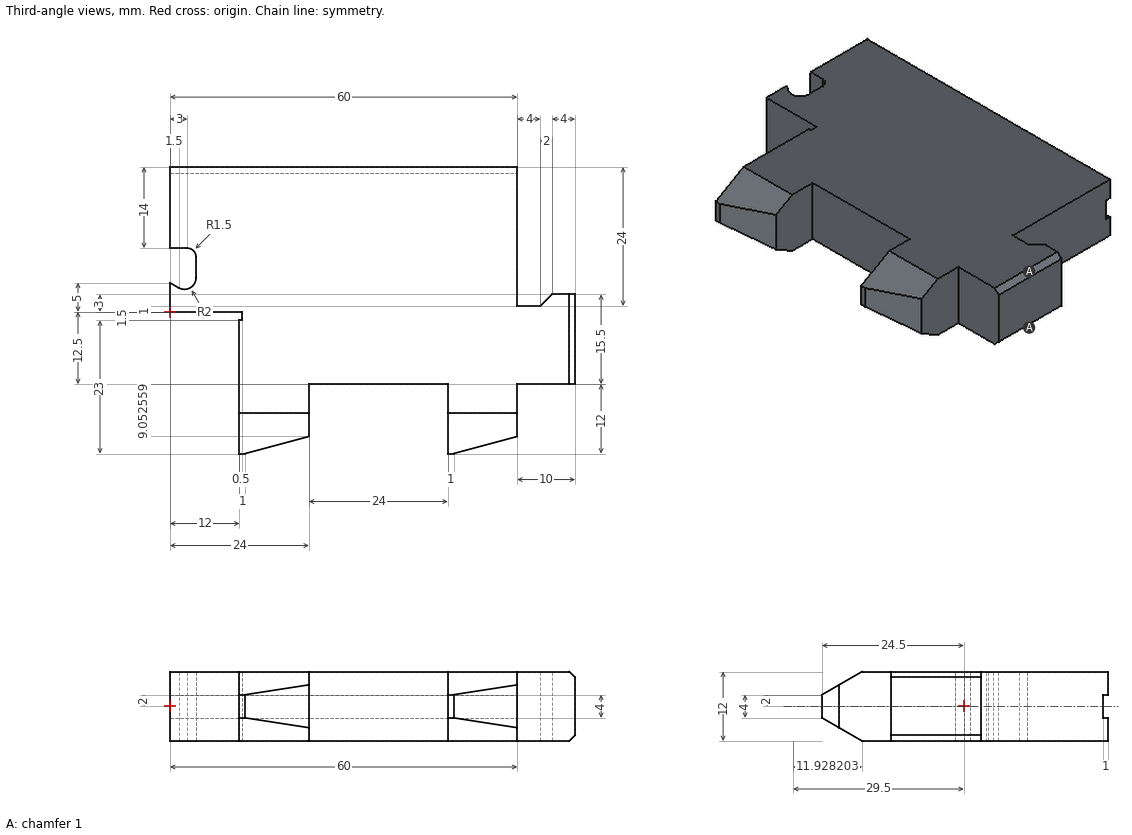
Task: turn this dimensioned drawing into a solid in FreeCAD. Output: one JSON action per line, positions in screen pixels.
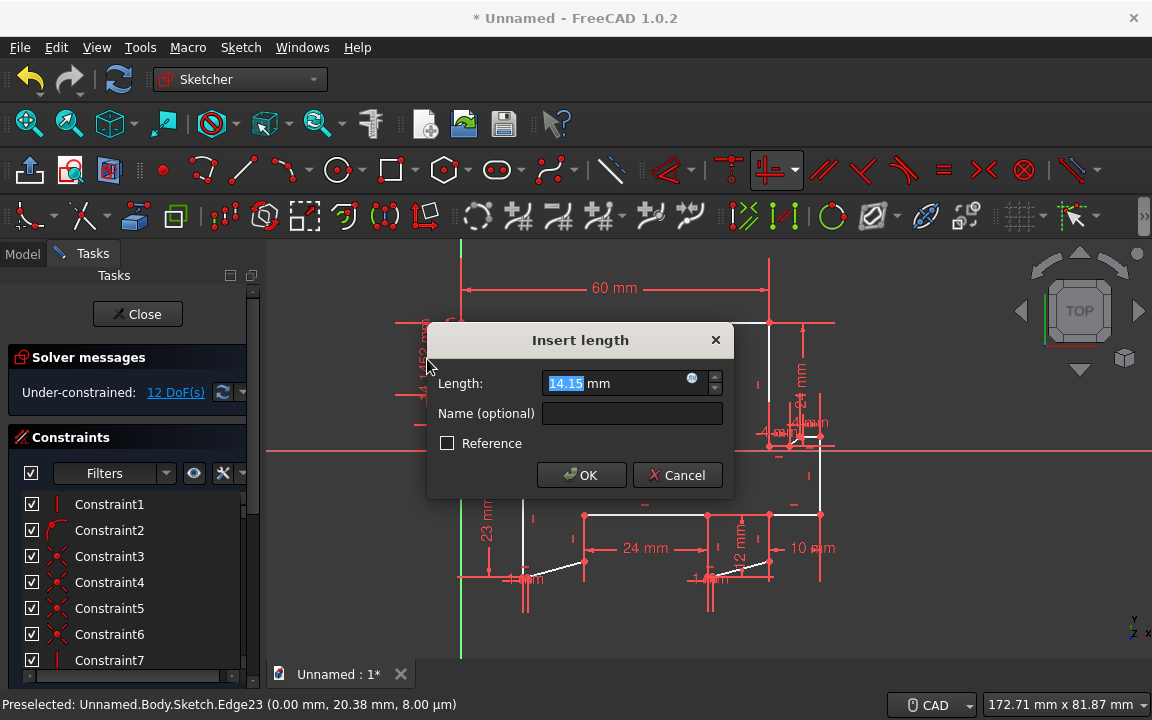
{"action": "type", "text": "14"}
{"action": "key", "text": "Return"}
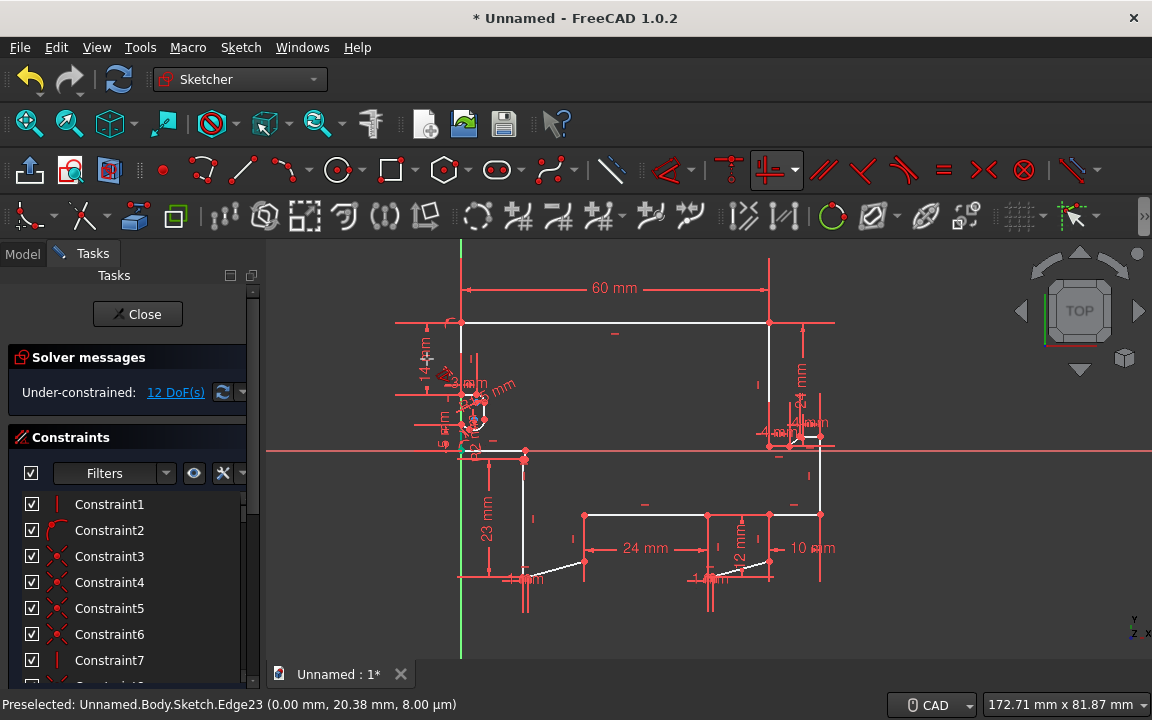
{"action": "scroll", "coordinate": [820, 437], "scroll_direction": "up", "scroll_amount": 5}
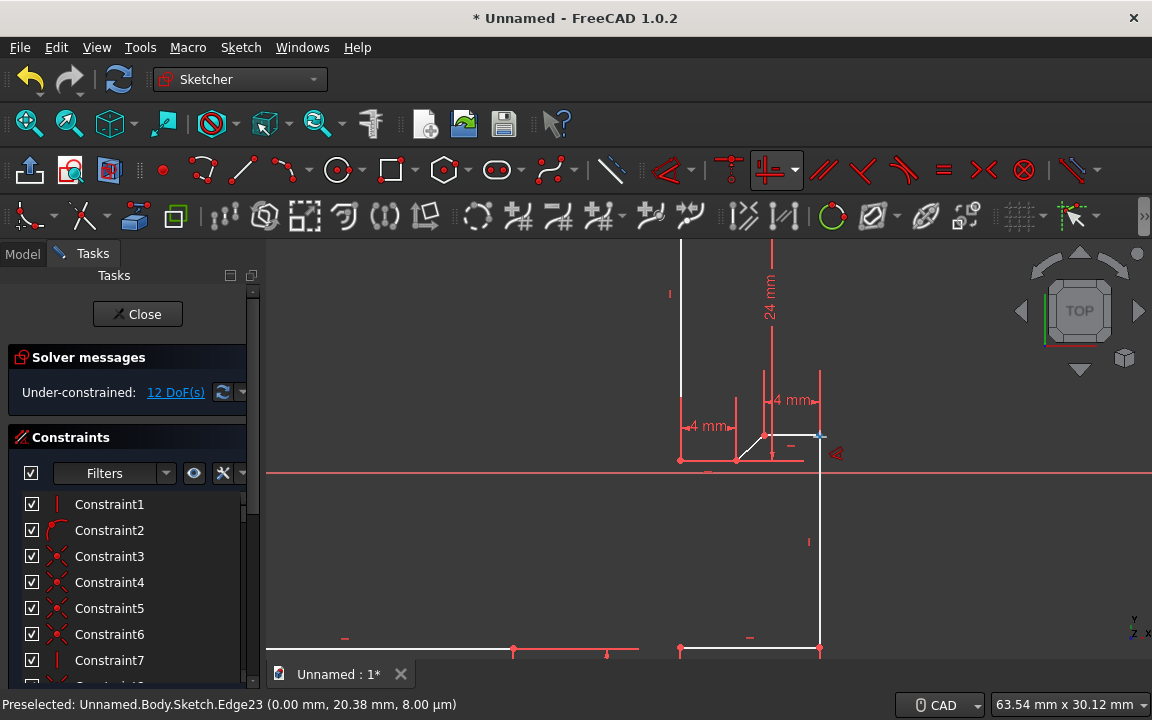
{"action": "left_click", "coordinate": [820, 435]}
{"action": "left_click", "coordinate": [854, 454]}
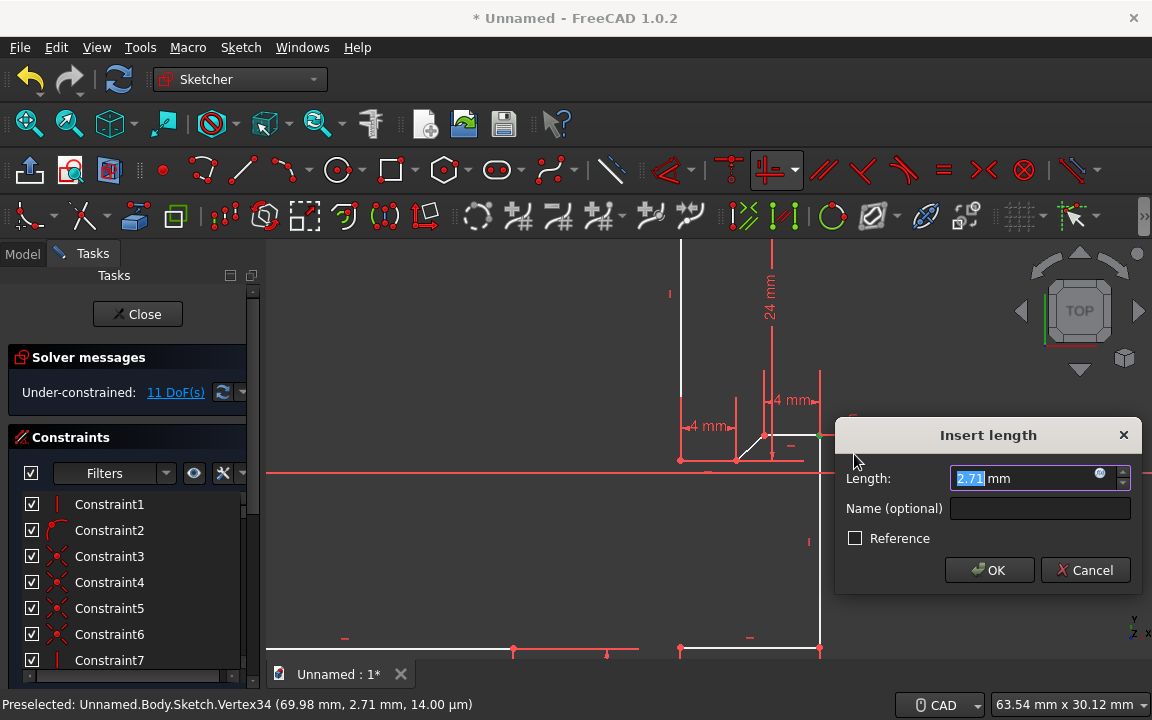
{"action": "type", "text": "3"}
{"action": "key", "text": "Return"}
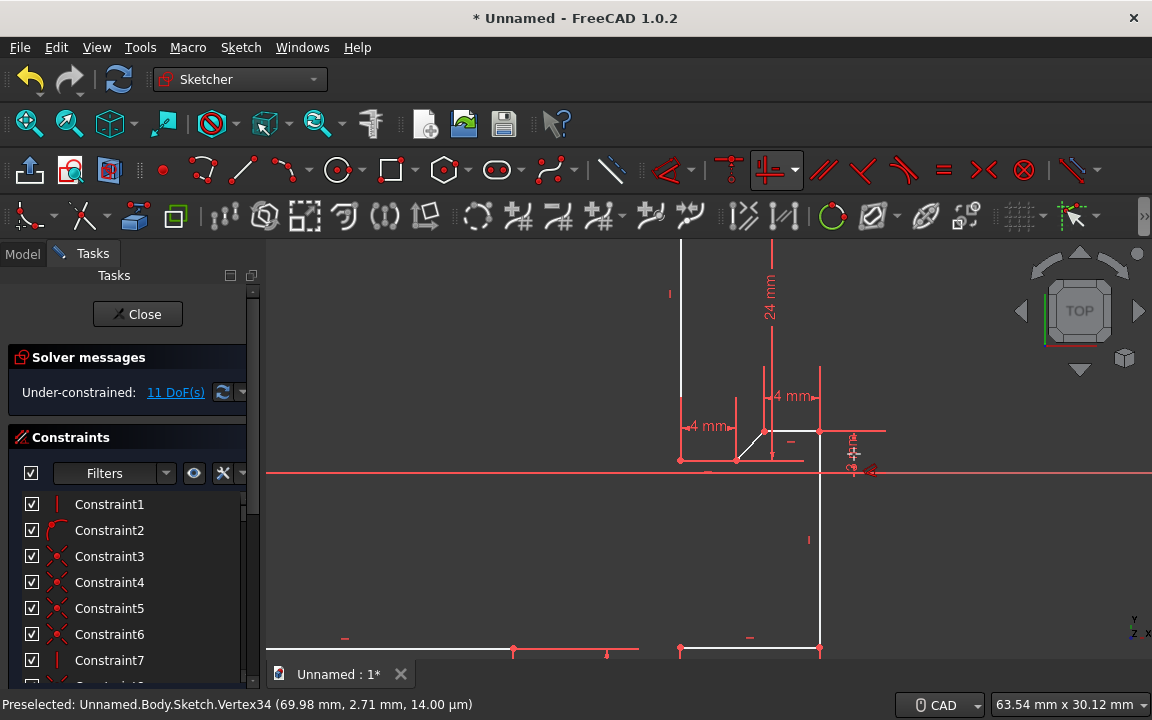
{"action": "scroll", "coordinate": [736, 461], "scroll_direction": "up", "scroll_amount": 6}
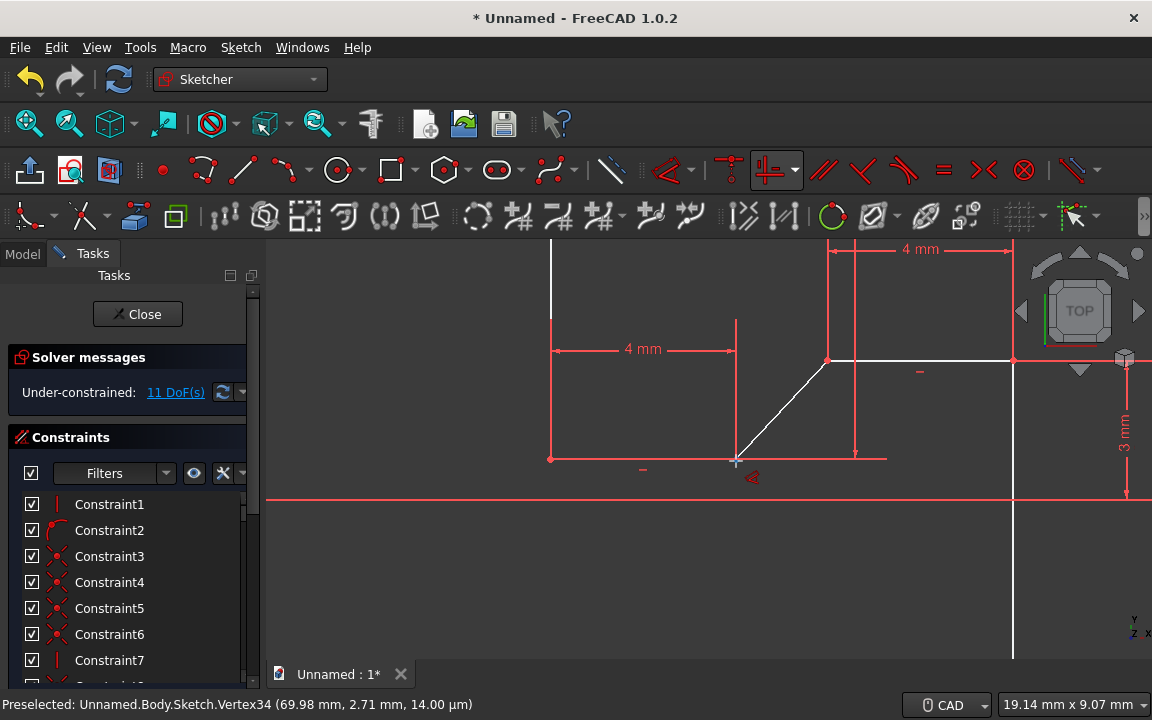
{"action": "left_click", "coordinate": [736, 459]}
{"action": "left_click", "coordinate": [770, 479]}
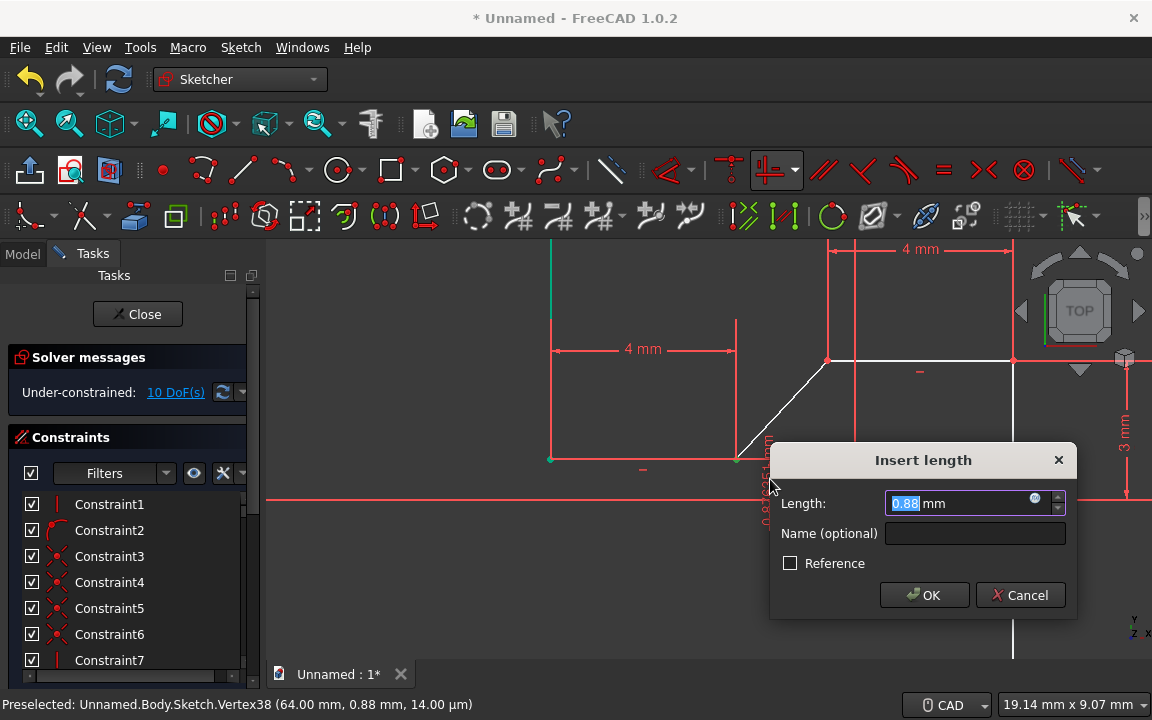
{"action": "type", "text": "1"}
{"action": "key", "text": "Return"}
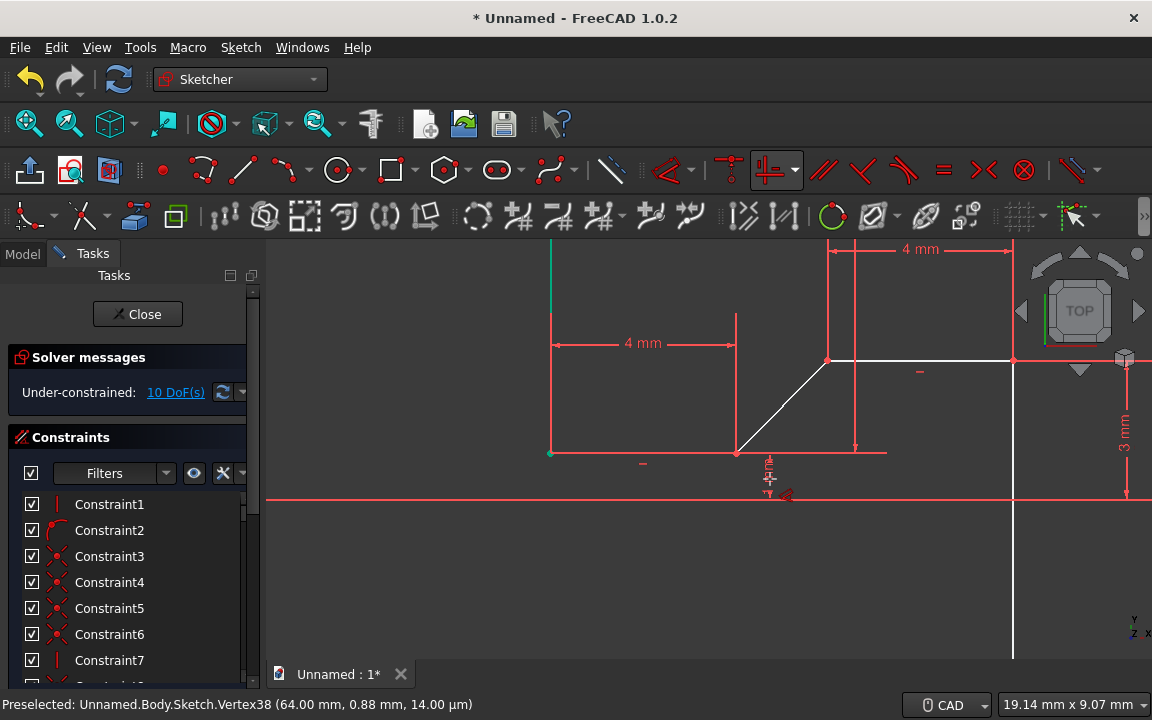
{"action": "left_click", "coordinate": [800, 389]}
{"action": "left_click", "coordinate": [782, 327]}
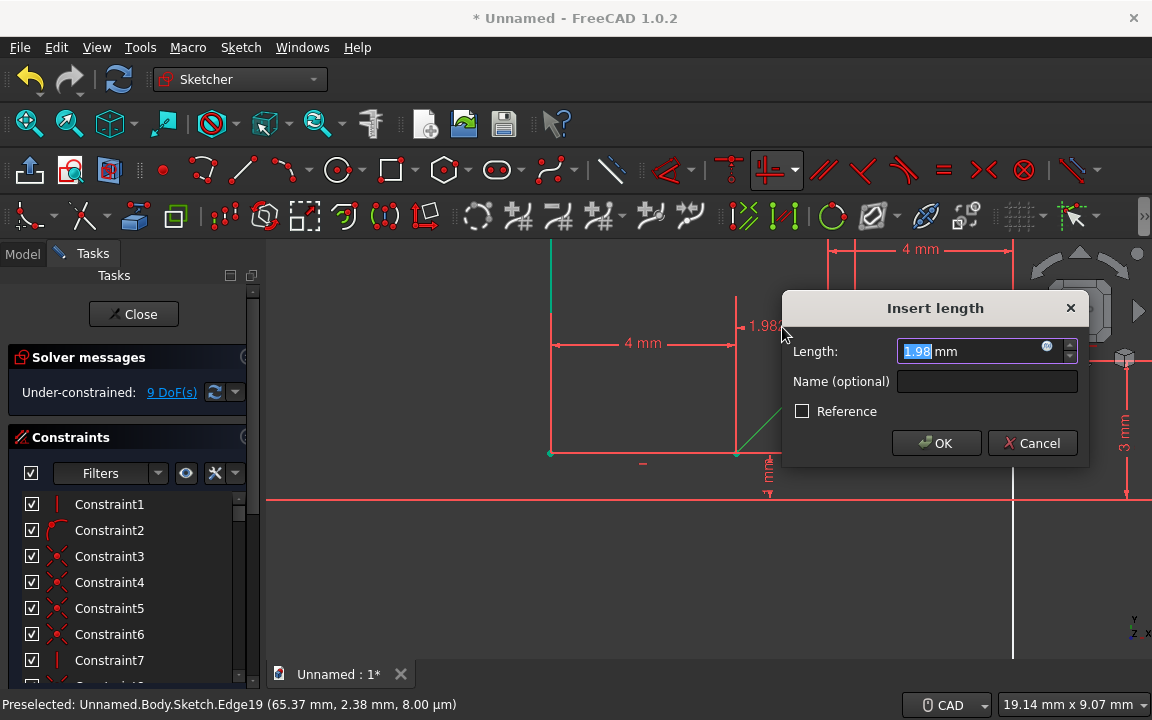
{"action": "type", "text": "2"}
{"action": "key", "text": "Return"}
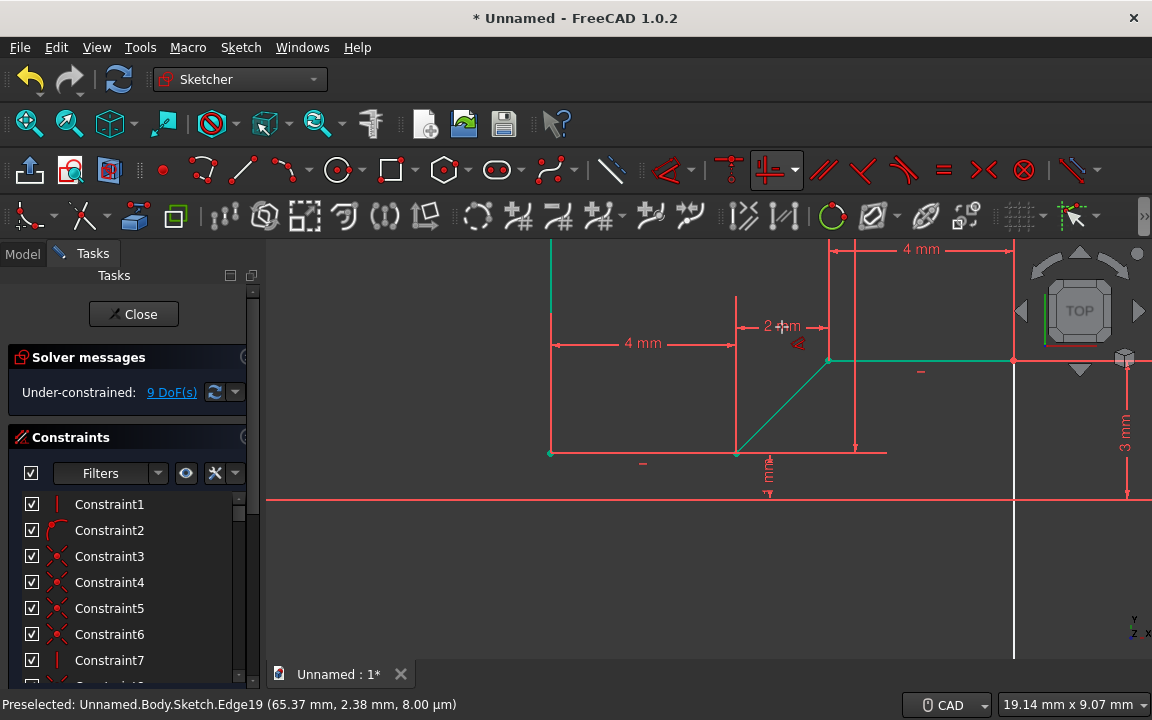
{"action": "scroll", "coordinate": [796, 444], "scroll_direction": "down", "scroll_amount": 11}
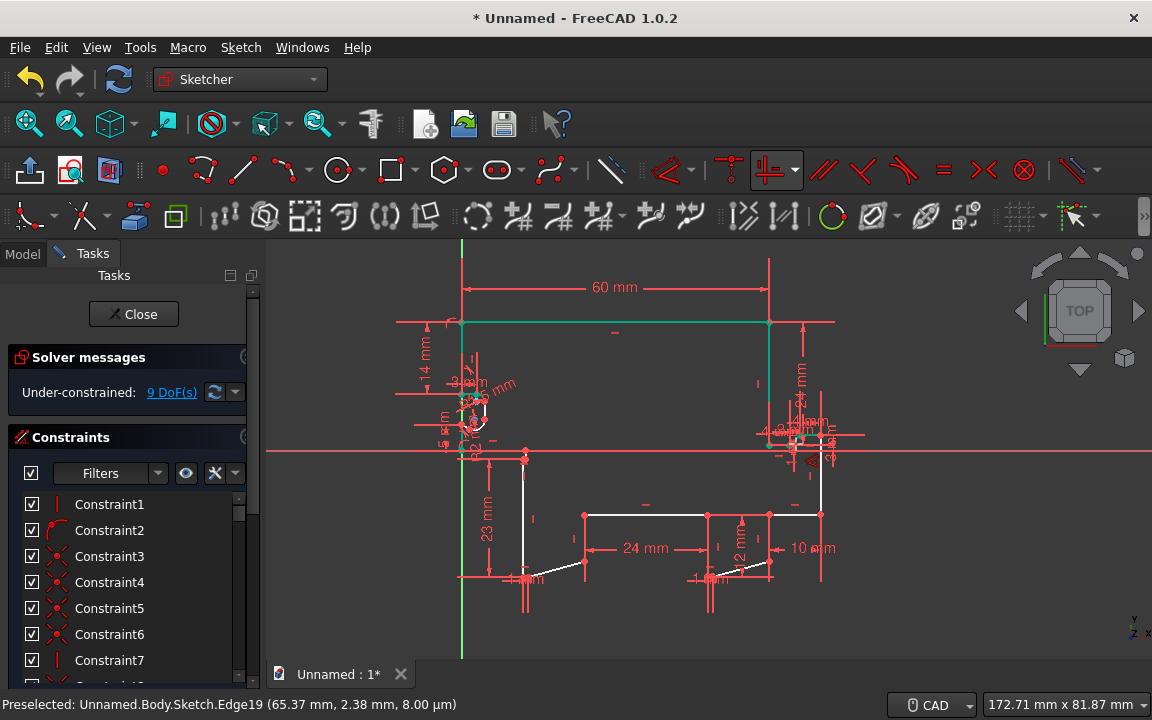
{"action": "scroll", "coordinate": [526, 453], "scroll_direction": "up", "scroll_amount": 9}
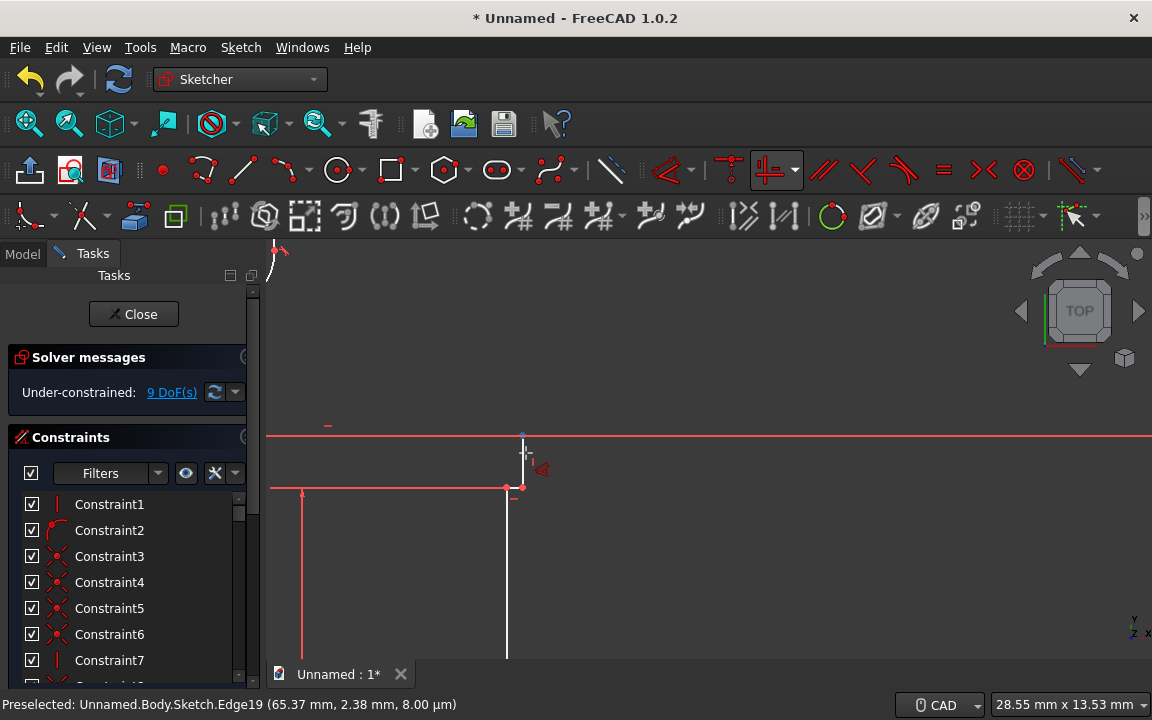
{"action": "left_click", "coordinate": [523, 451]}
{"action": "left_click", "coordinate": [489, 462]}